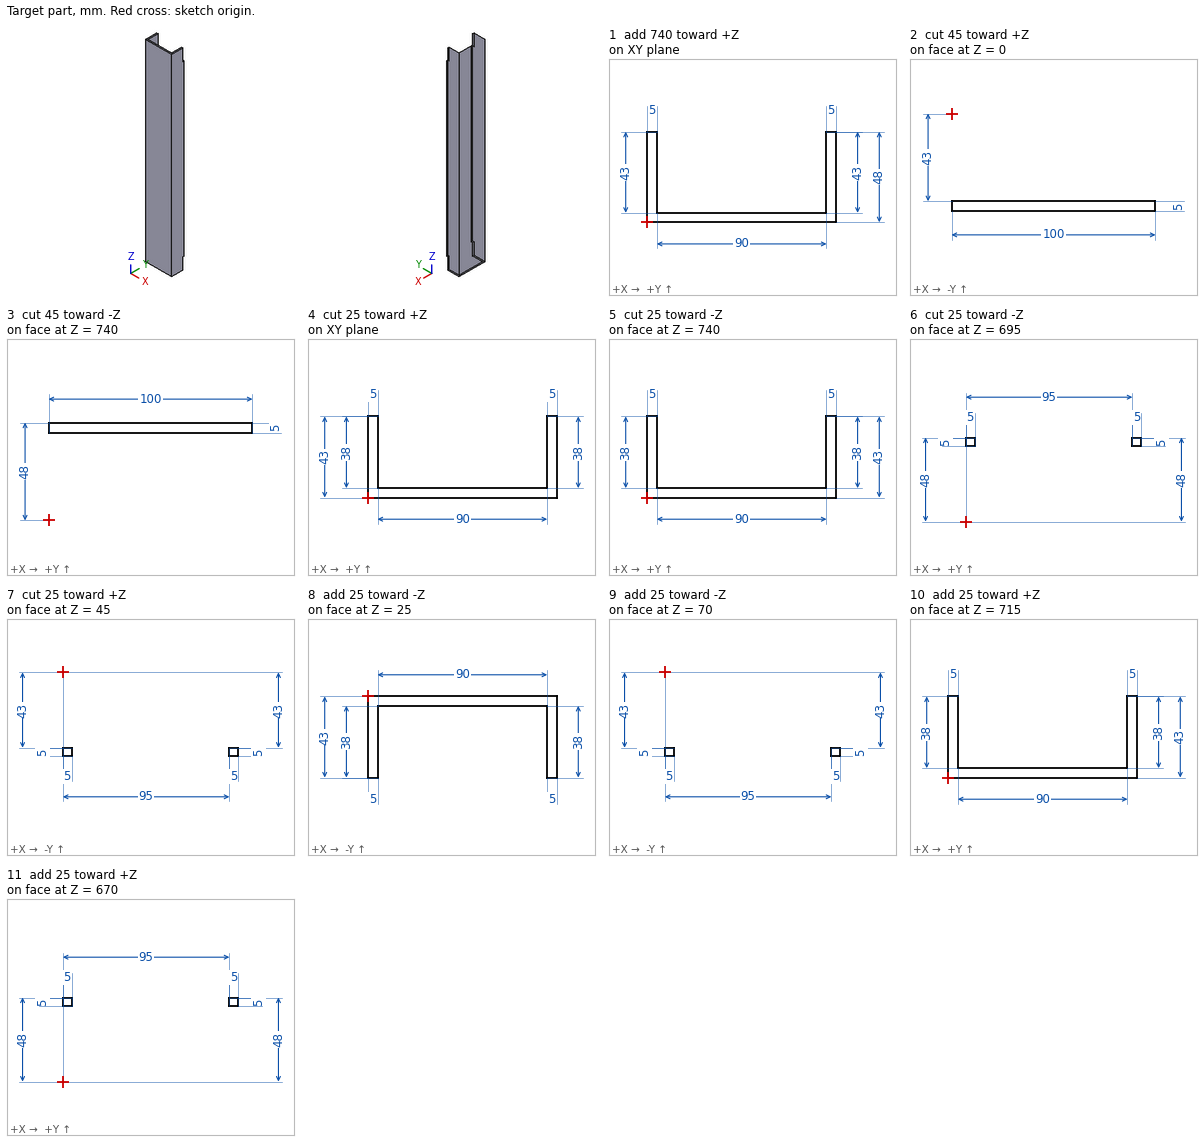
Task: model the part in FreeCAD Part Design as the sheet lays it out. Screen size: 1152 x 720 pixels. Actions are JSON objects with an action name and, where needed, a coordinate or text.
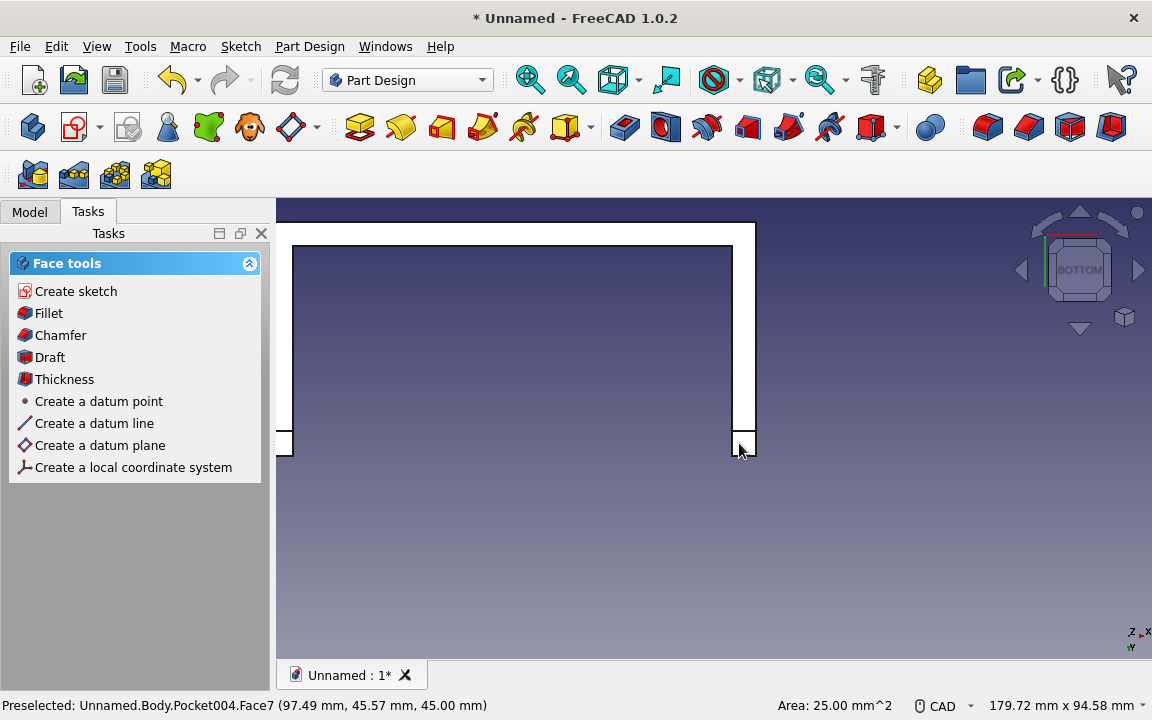
{"action": "left_click", "coordinate": [74, 128]}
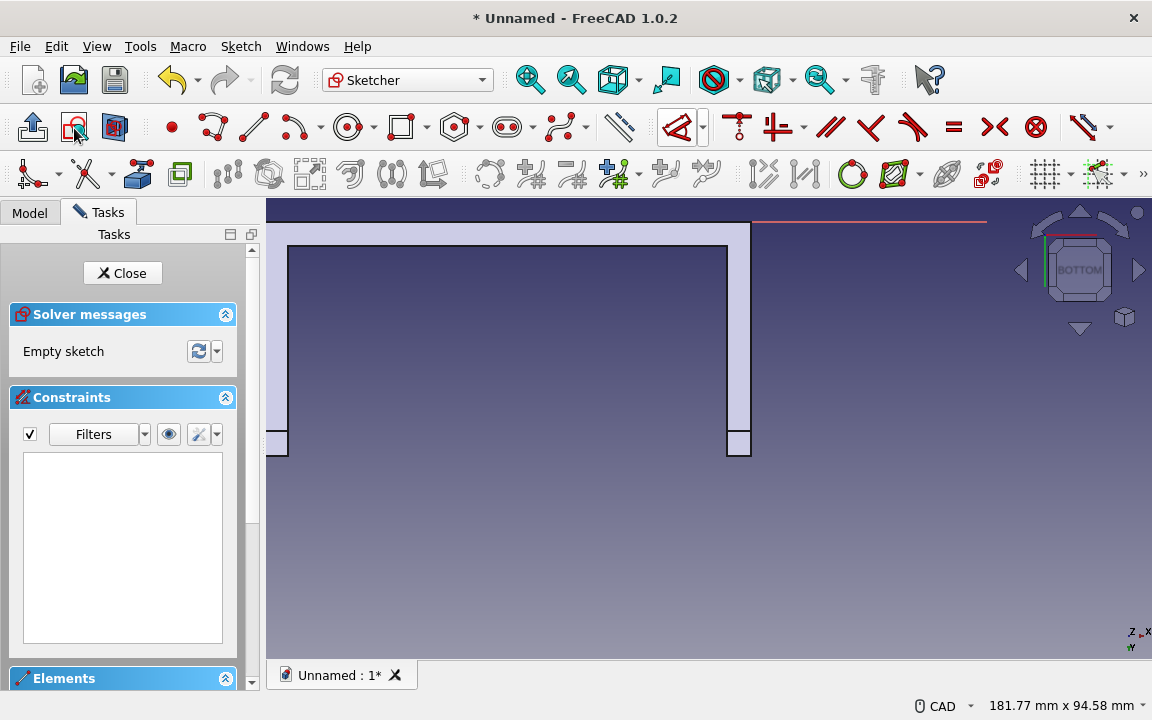
{"action": "scroll", "coordinate": [987, 631], "scroll_direction": "down", "scroll_amount": 1}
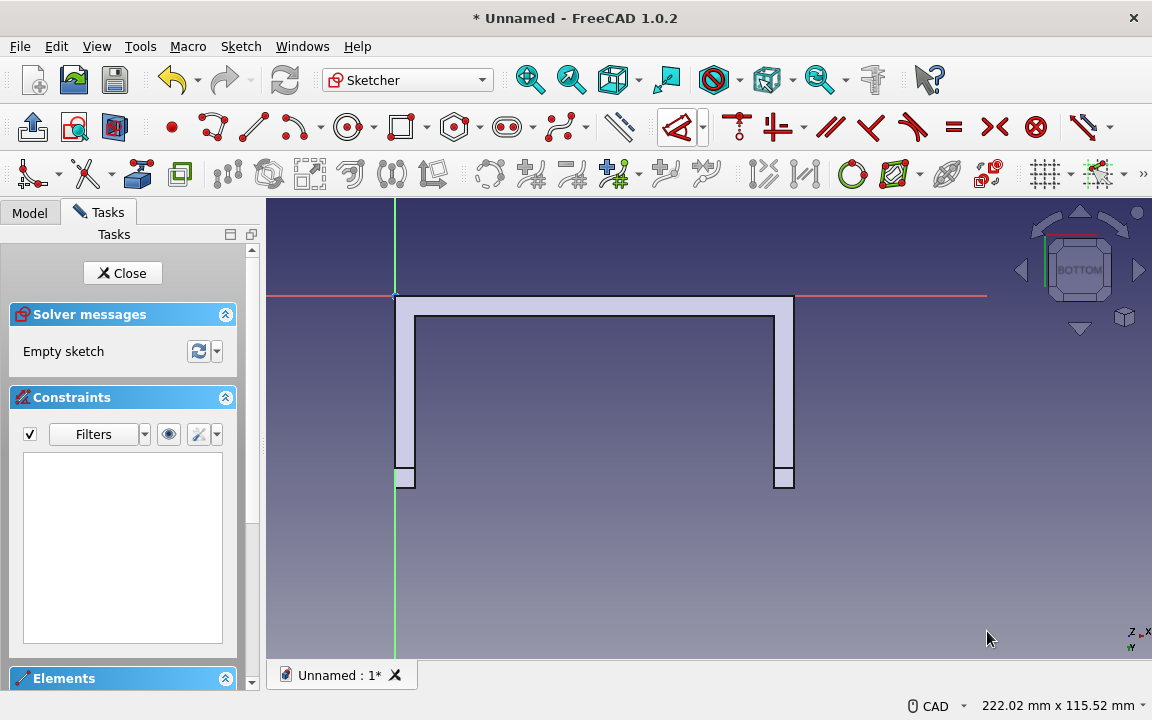
{"action": "left_click", "coordinate": [400, 128]}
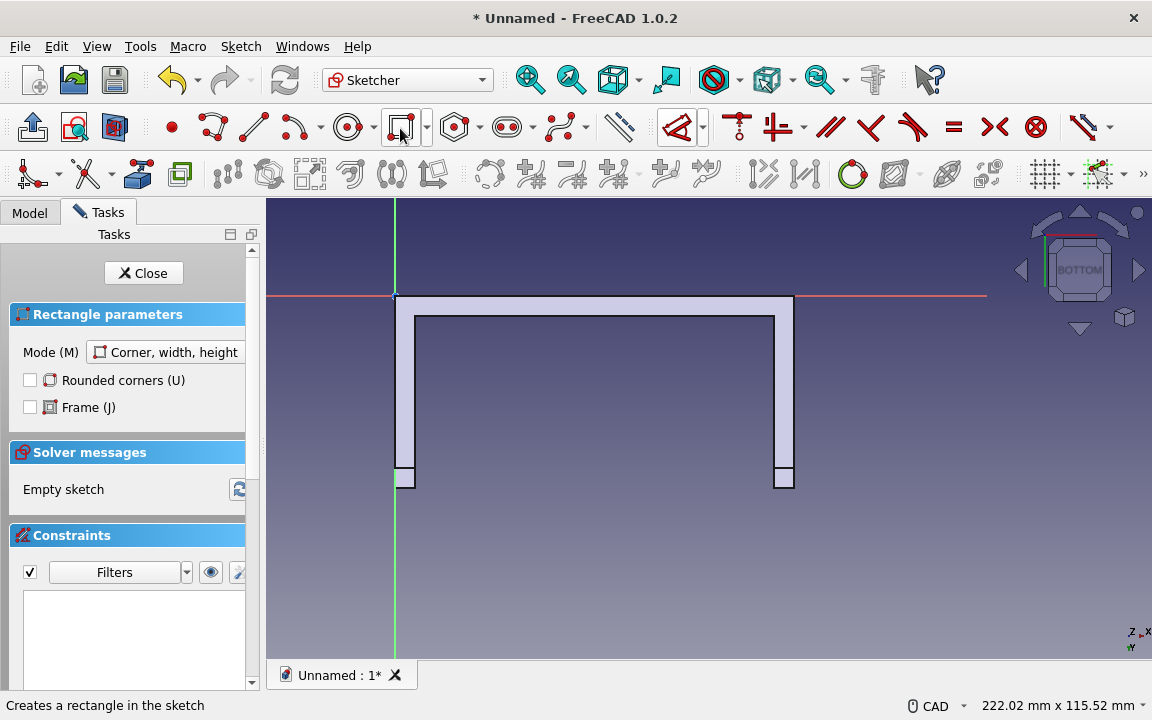
{"action": "left_click", "coordinate": [395, 468]}
{"action": "mouse_move", "coordinate": [415, 488]}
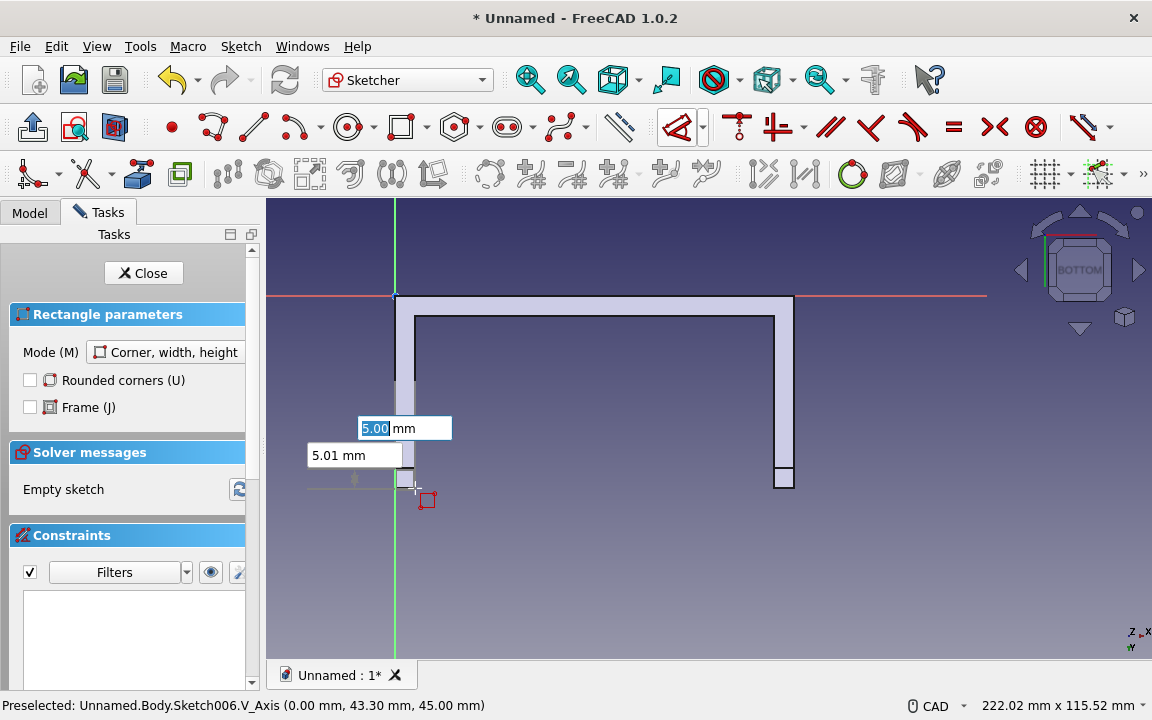
{"action": "type", "text": "5"}
{"action": "key", "text": "Tab"}
{"action": "type", "text": "5"}
{"action": "key", "text": "Return"}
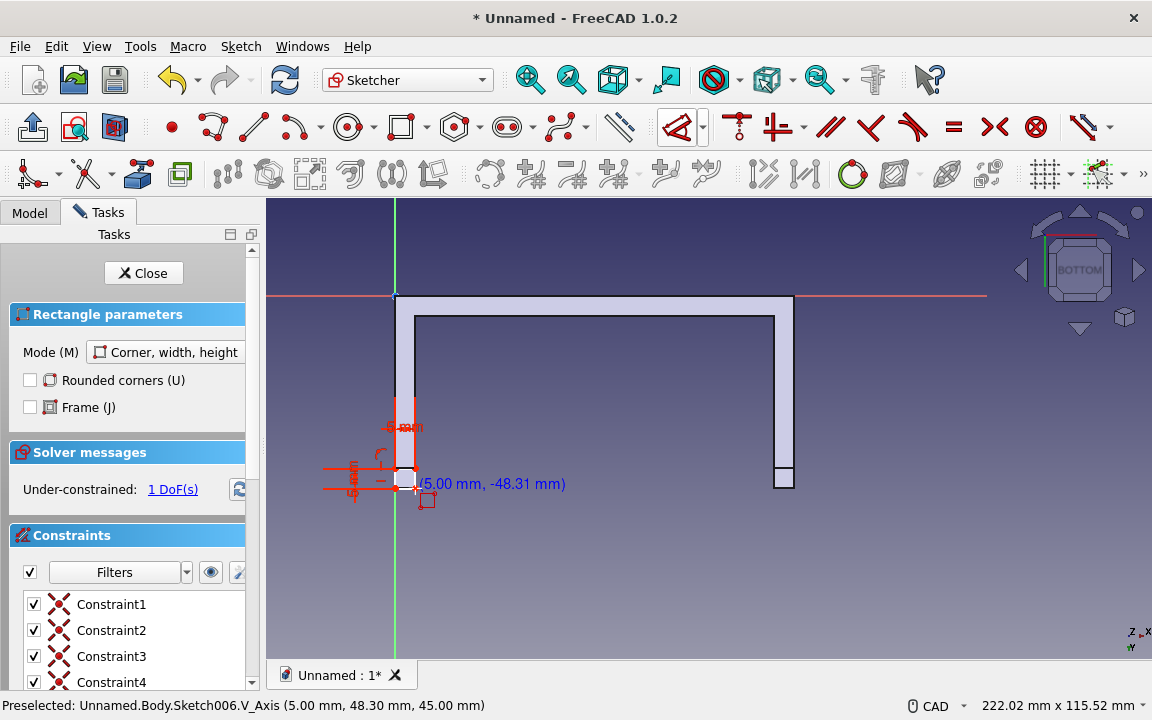
{"action": "left_click", "coordinate": [774, 468]}
{"action": "mouse_move", "coordinate": [794, 488]}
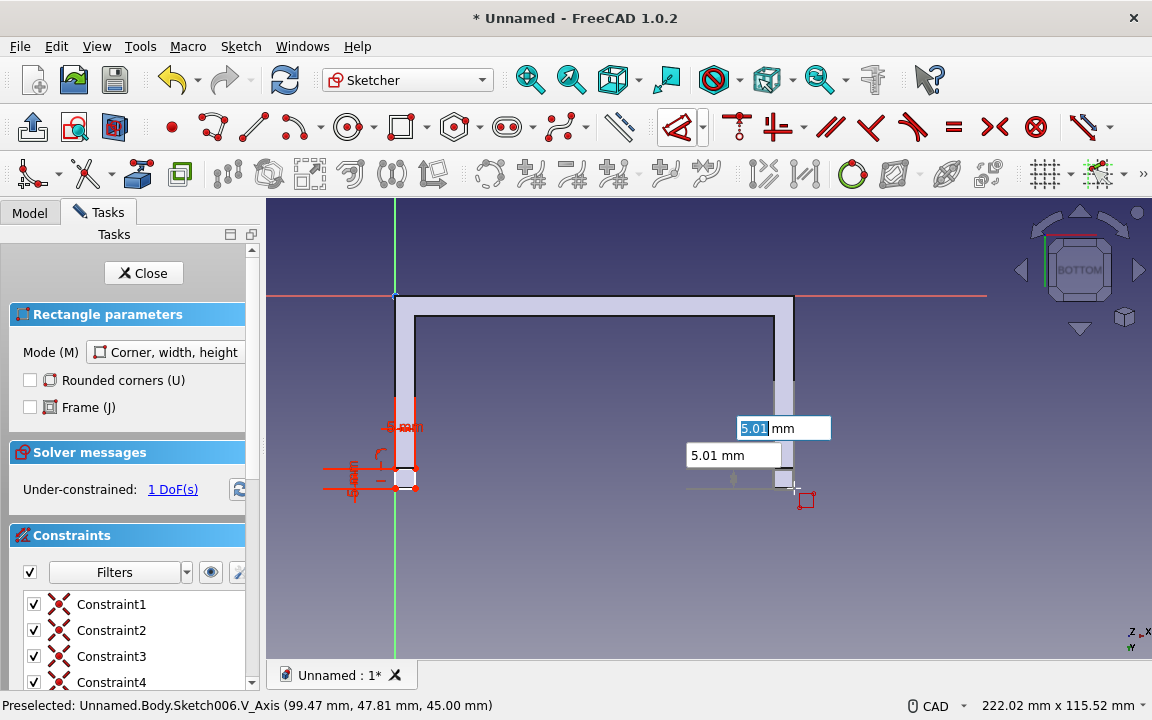
{"action": "type", "text": "5"}
{"action": "key", "text": "Tab"}
{"action": "type", "text": "5"}
{"action": "key", "text": "Return"}
{"action": "key", "text": "Escape"}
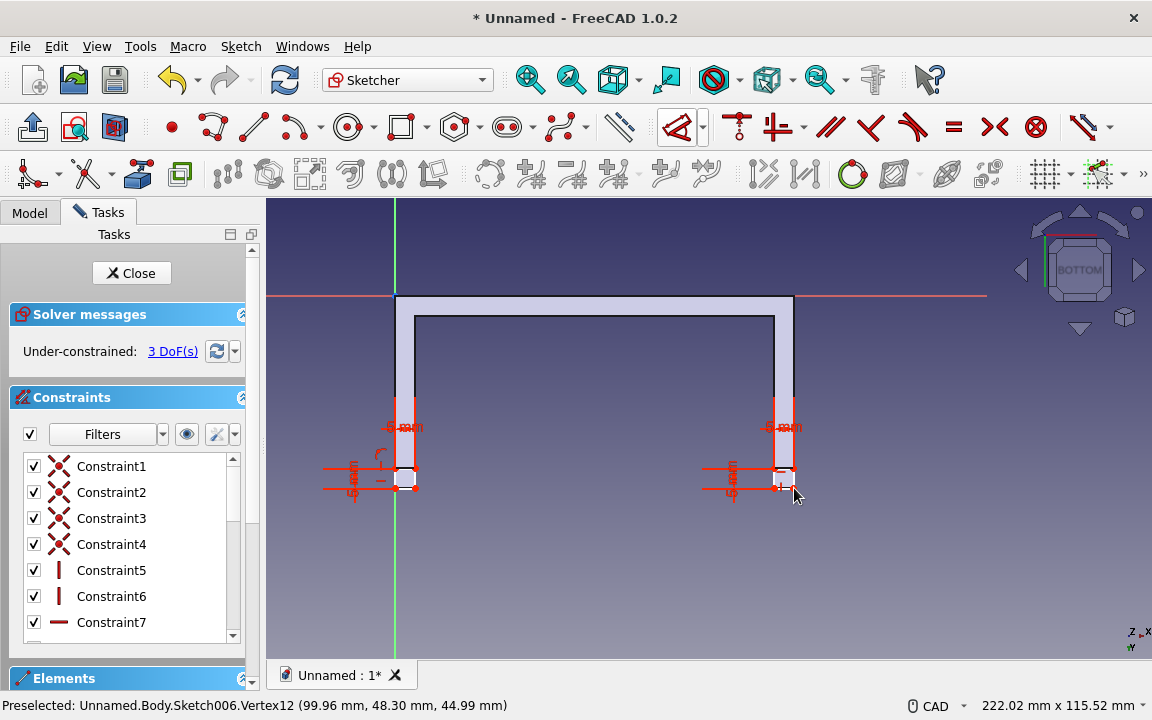
{"action": "left_click", "coordinate": [395, 469]}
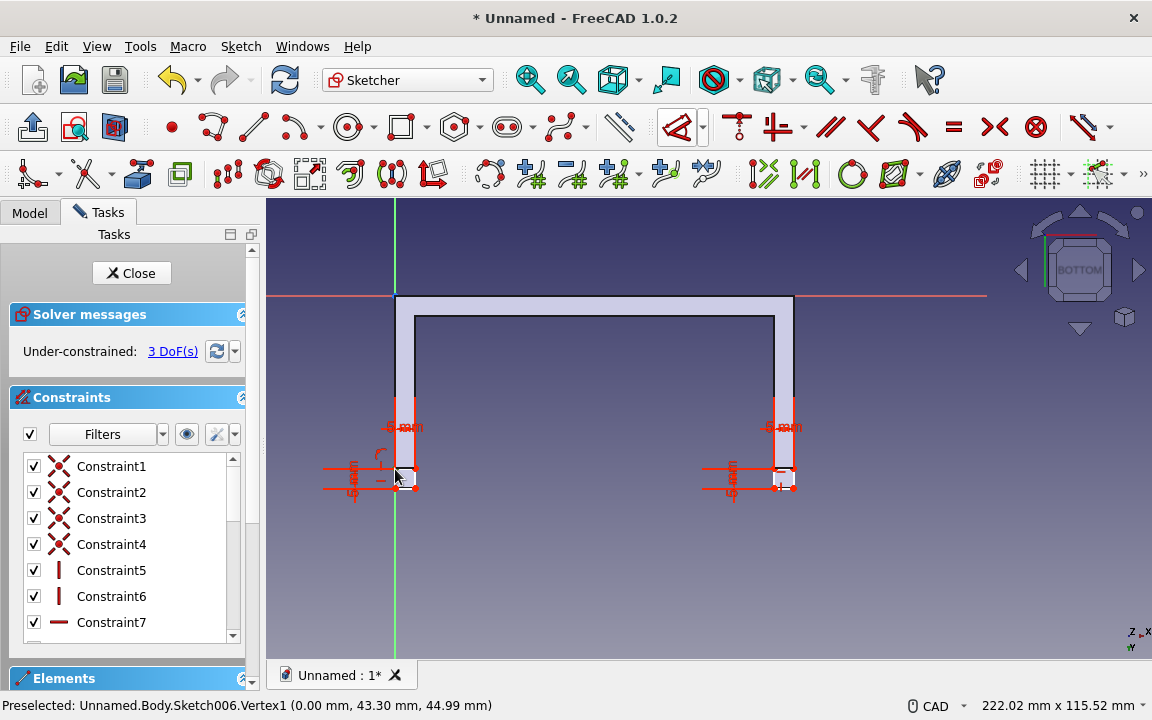
{"action": "key", "text": "i"}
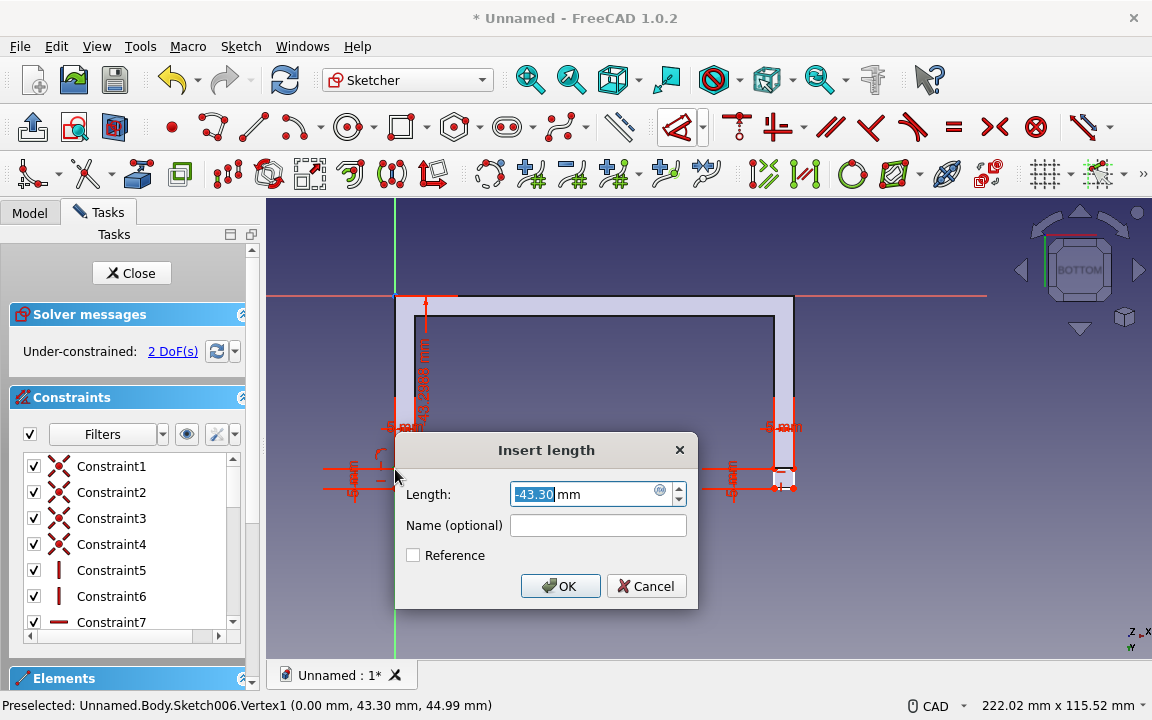
{"action": "type", "text": "-43"}
{"action": "key", "text": "Return"}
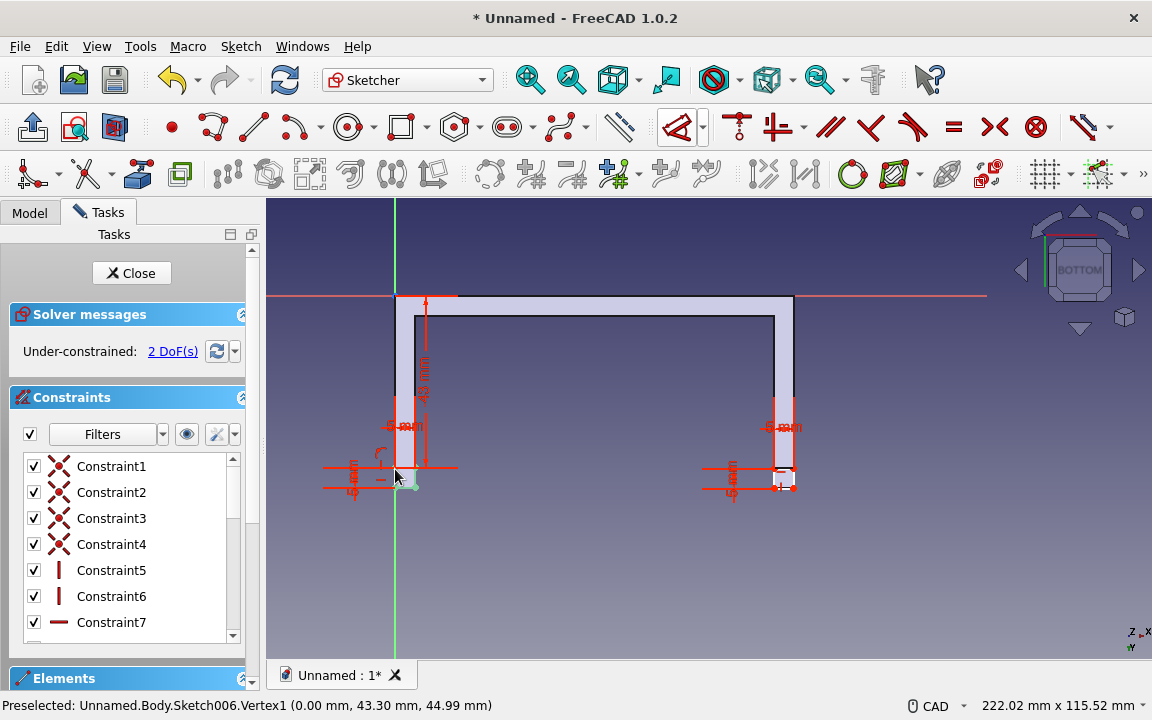
{"action": "left_click", "coordinate": [774, 469]}